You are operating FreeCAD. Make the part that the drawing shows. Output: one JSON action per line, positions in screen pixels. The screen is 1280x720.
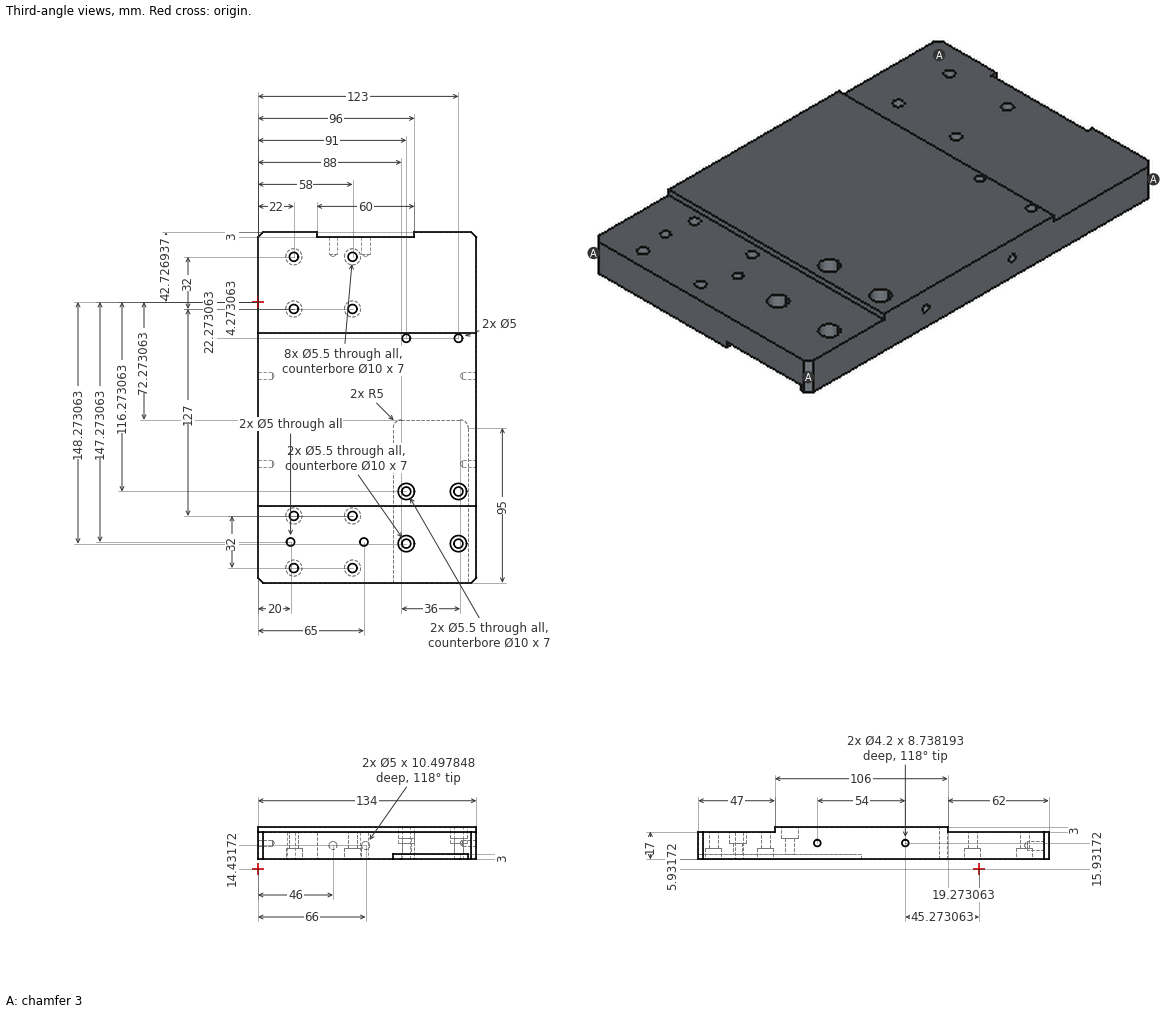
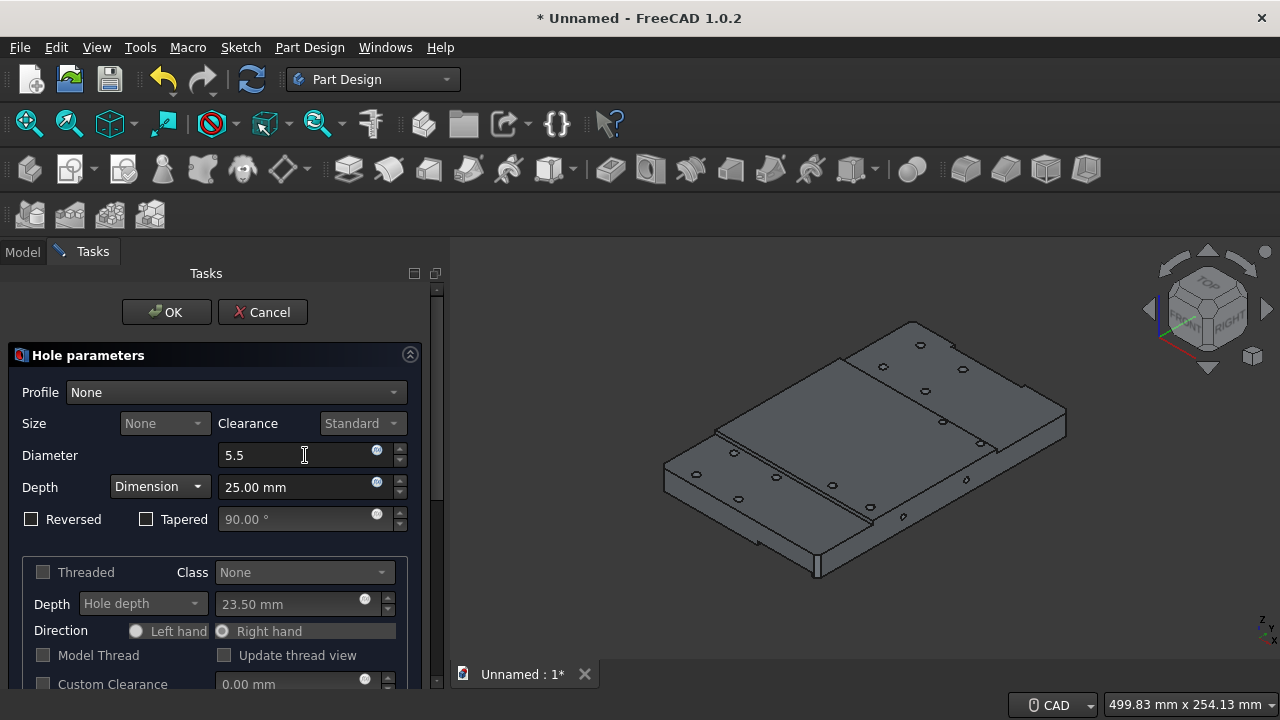
{"action": "left_click", "coordinate": [161, 486]}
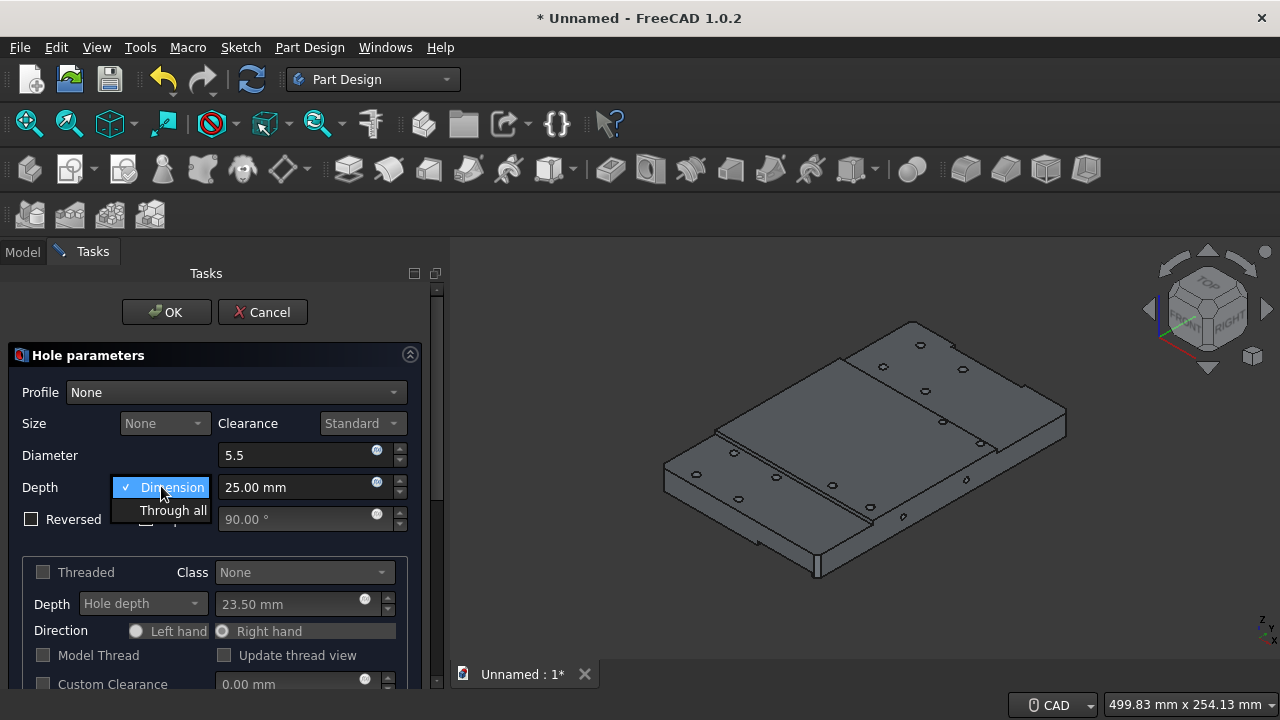
{"action": "left_click", "coordinate": [160, 510]}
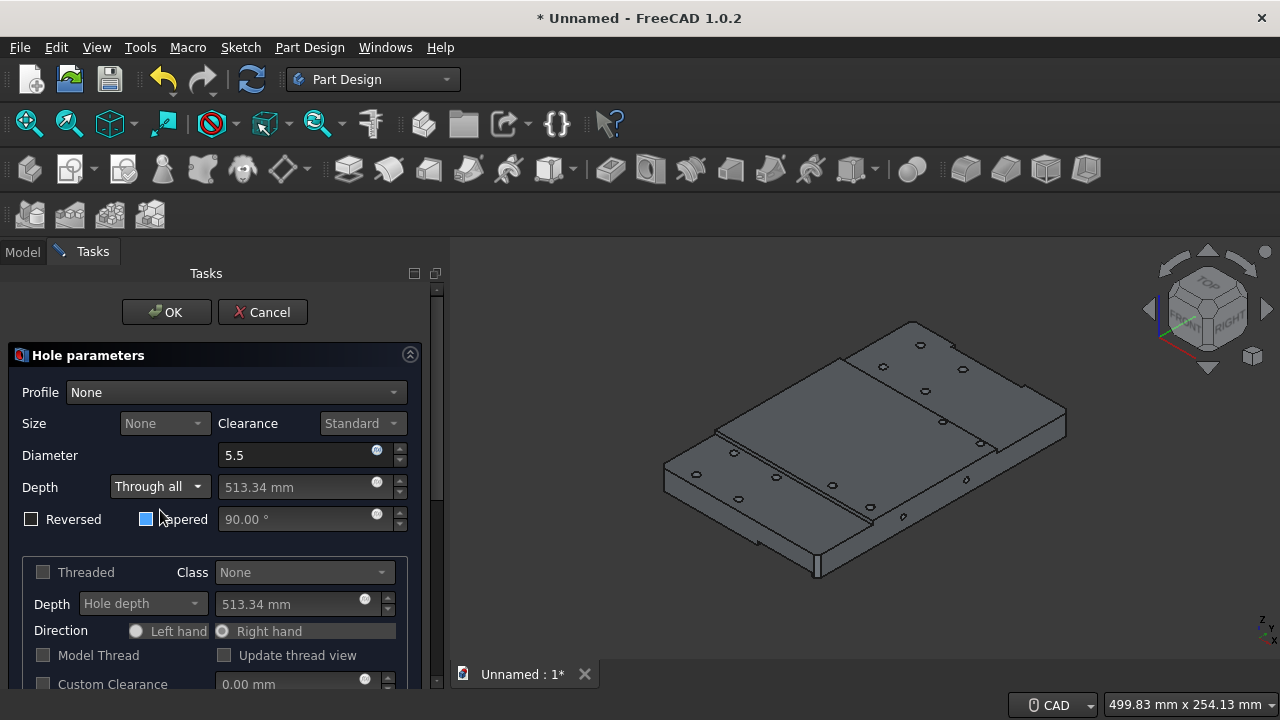
{"action": "scroll", "coordinate": [437, 486], "scroll_direction": "down", "scroll_amount": 3}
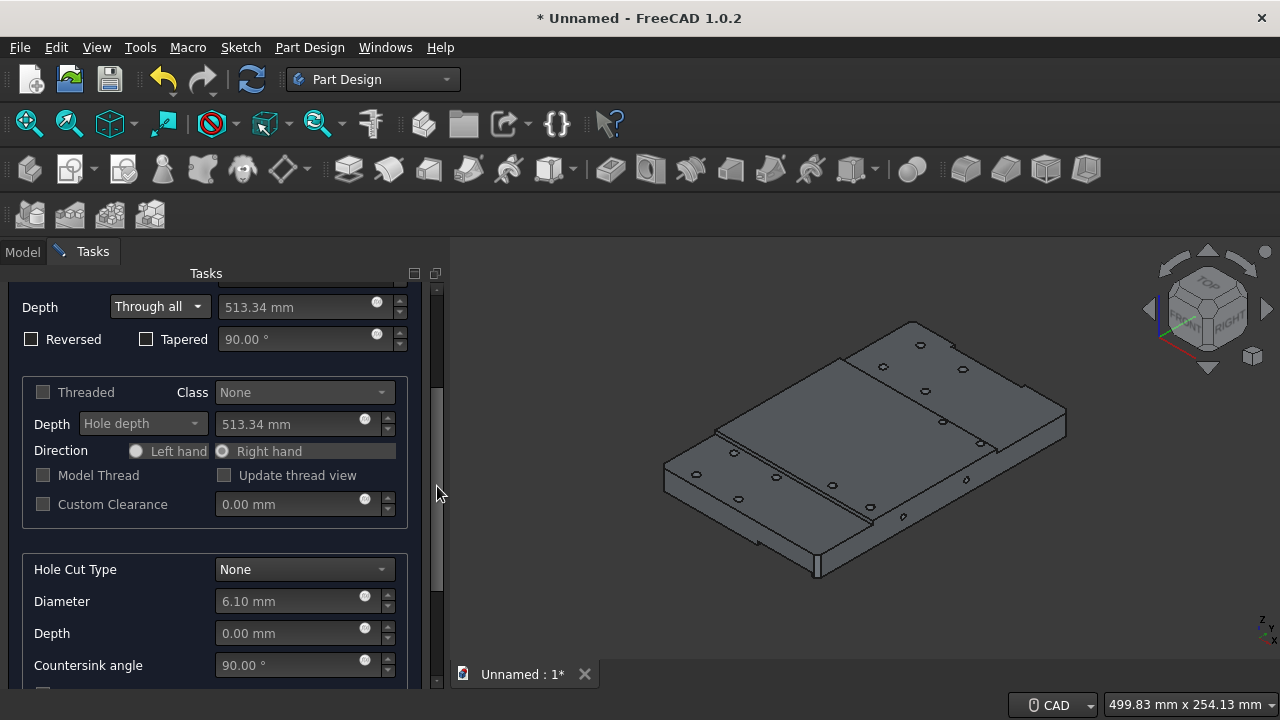
{"action": "left_click", "coordinate": [306, 570]}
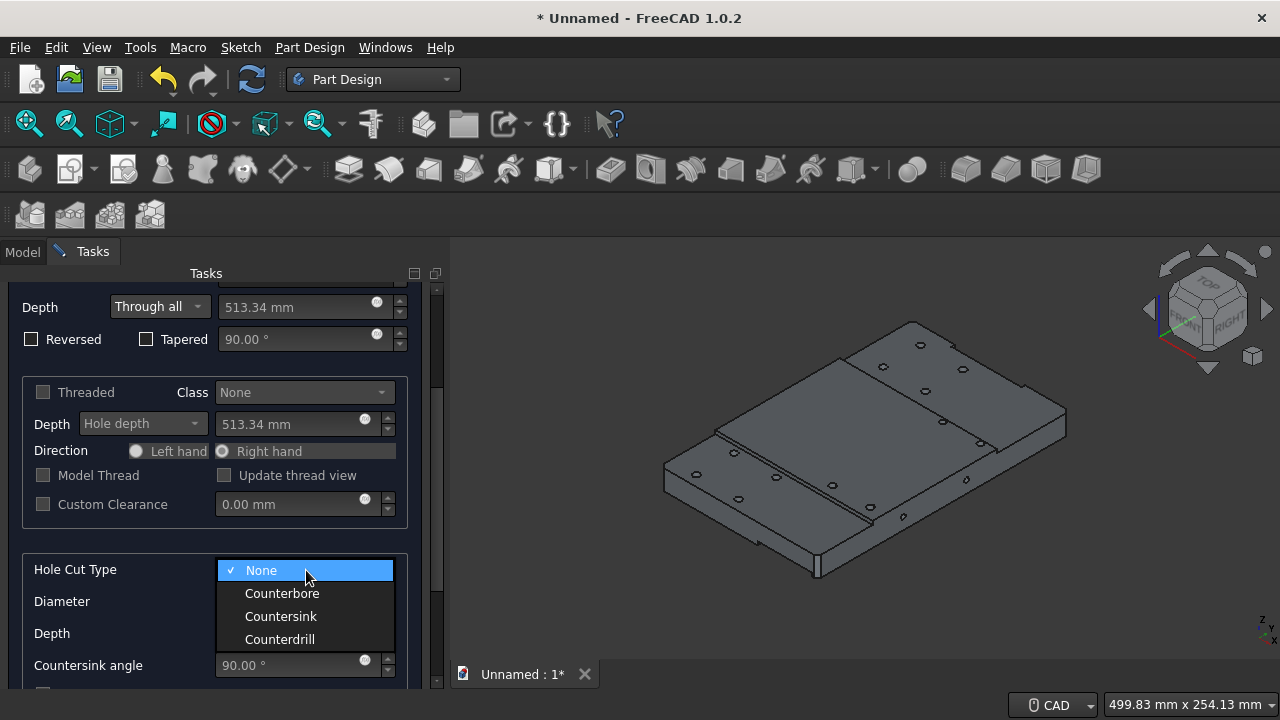
{"action": "left_click", "coordinate": [304, 594]}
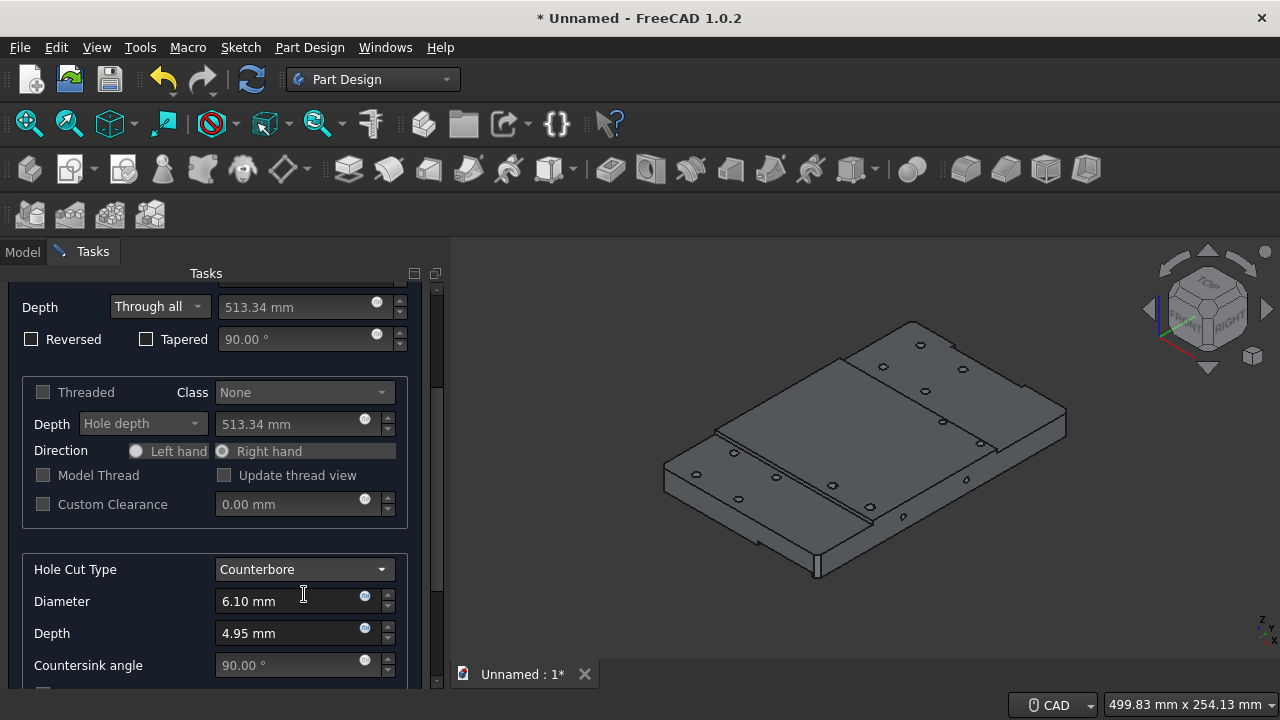
{"action": "triple_click", "coordinate": [298, 601]}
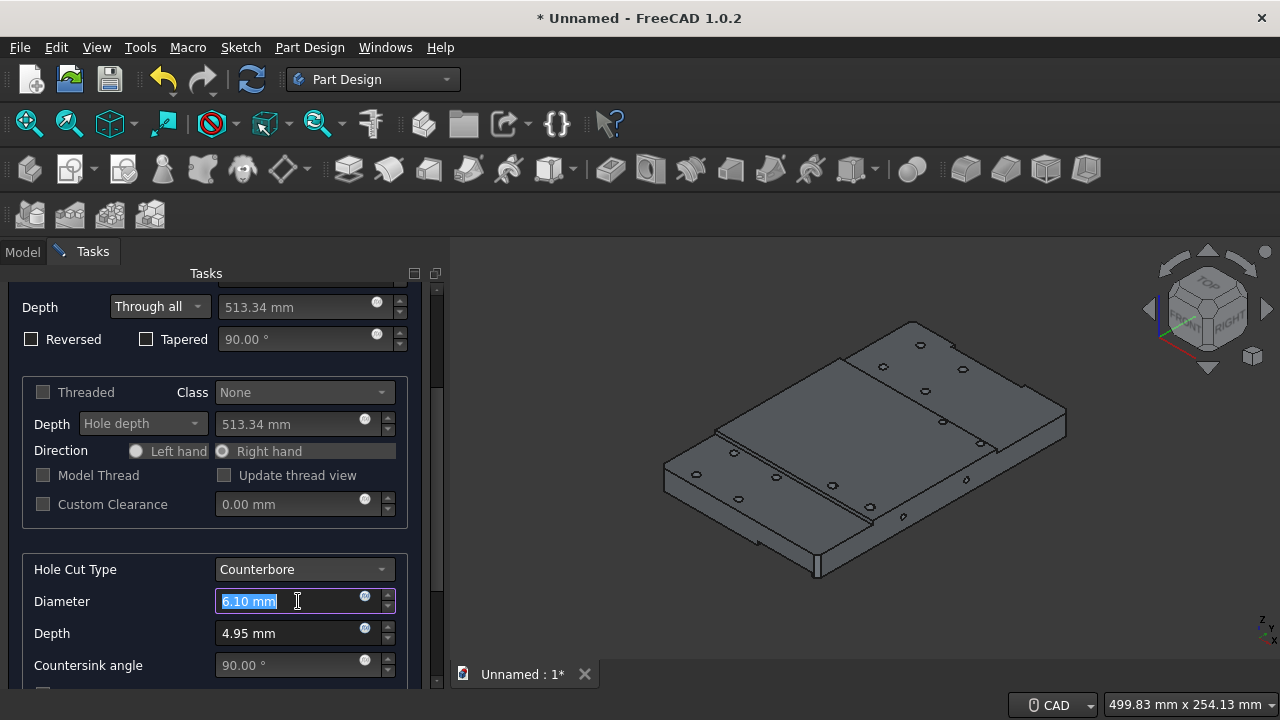
{"action": "type", "text": "10"}
{"action": "key", "text": "Tab"}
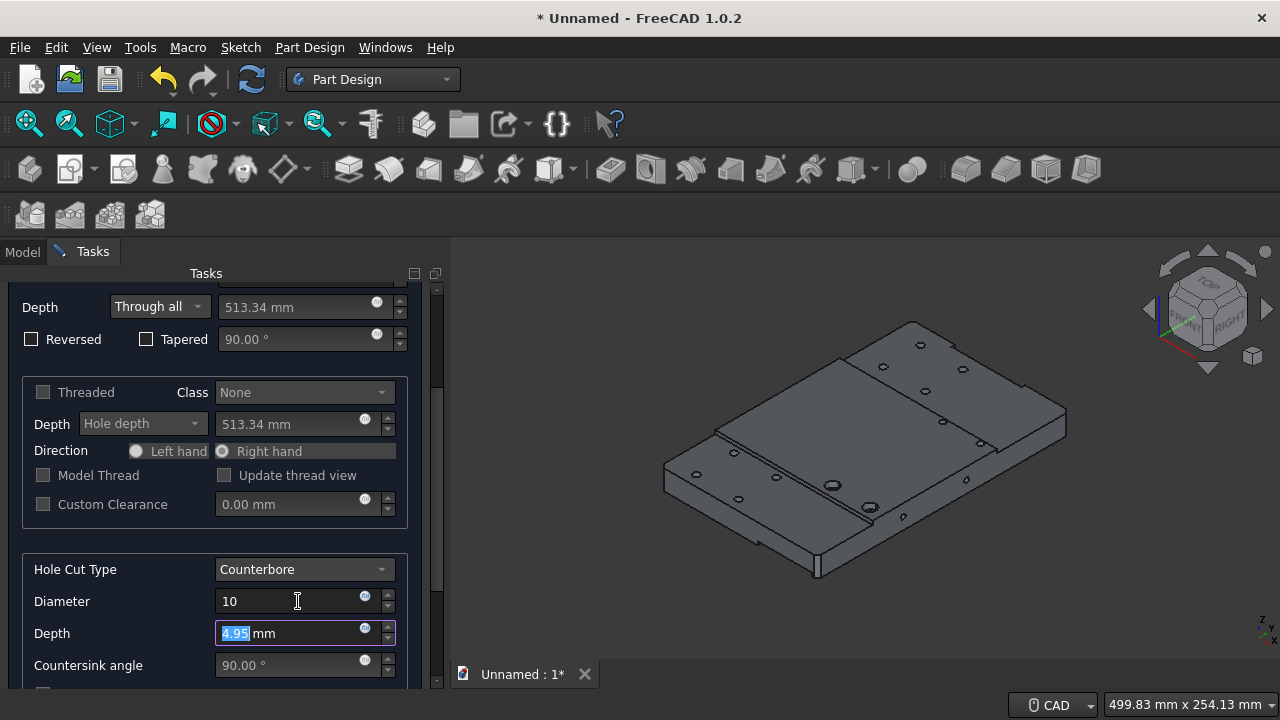
{"action": "type", "text": "7"}
{"action": "key", "text": "Tab"}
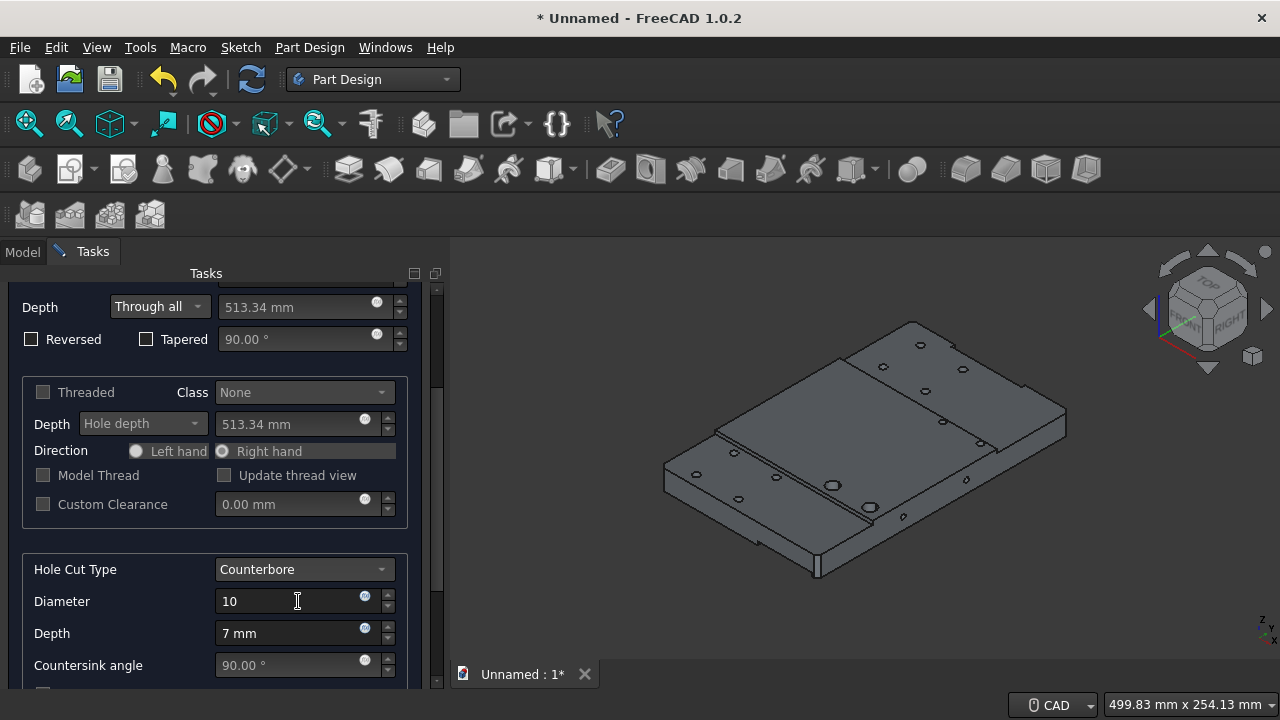
{"action": "scroll", "coordinate": [437, 486], "scroll_direction": "up", "scroll_amount": 4}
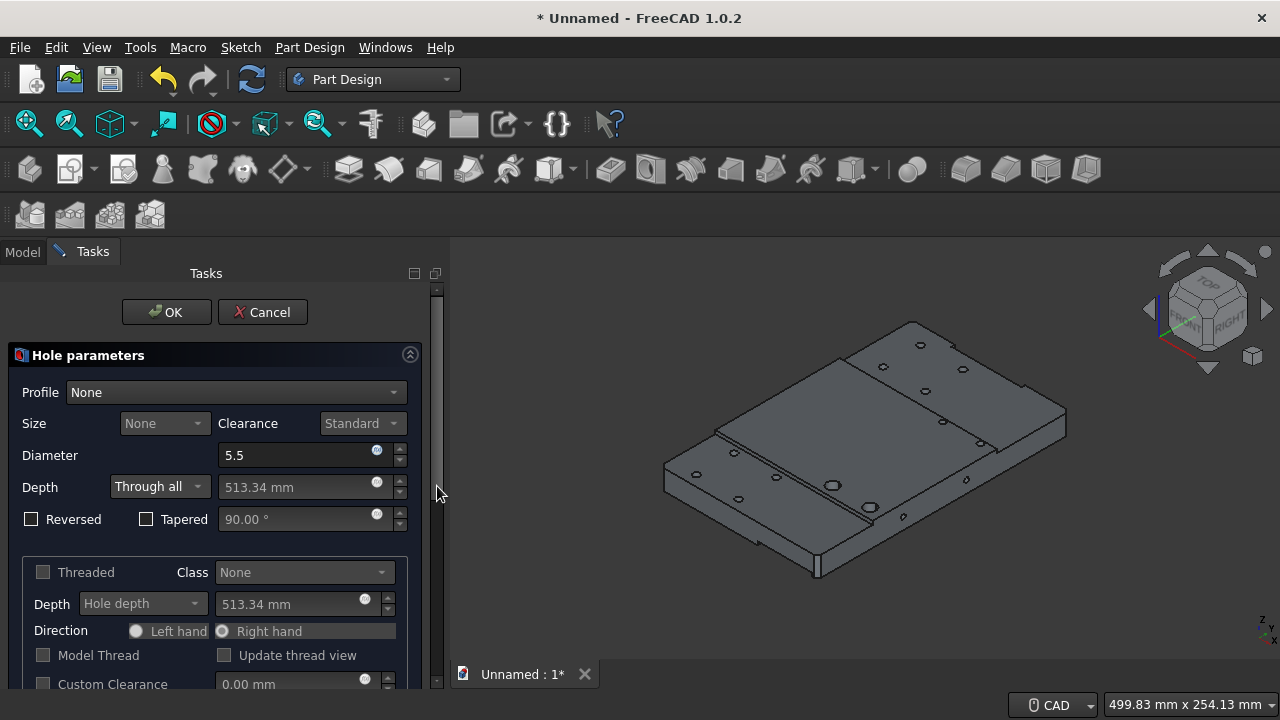
{"action": "left_click", "coordinate": [167, 312]}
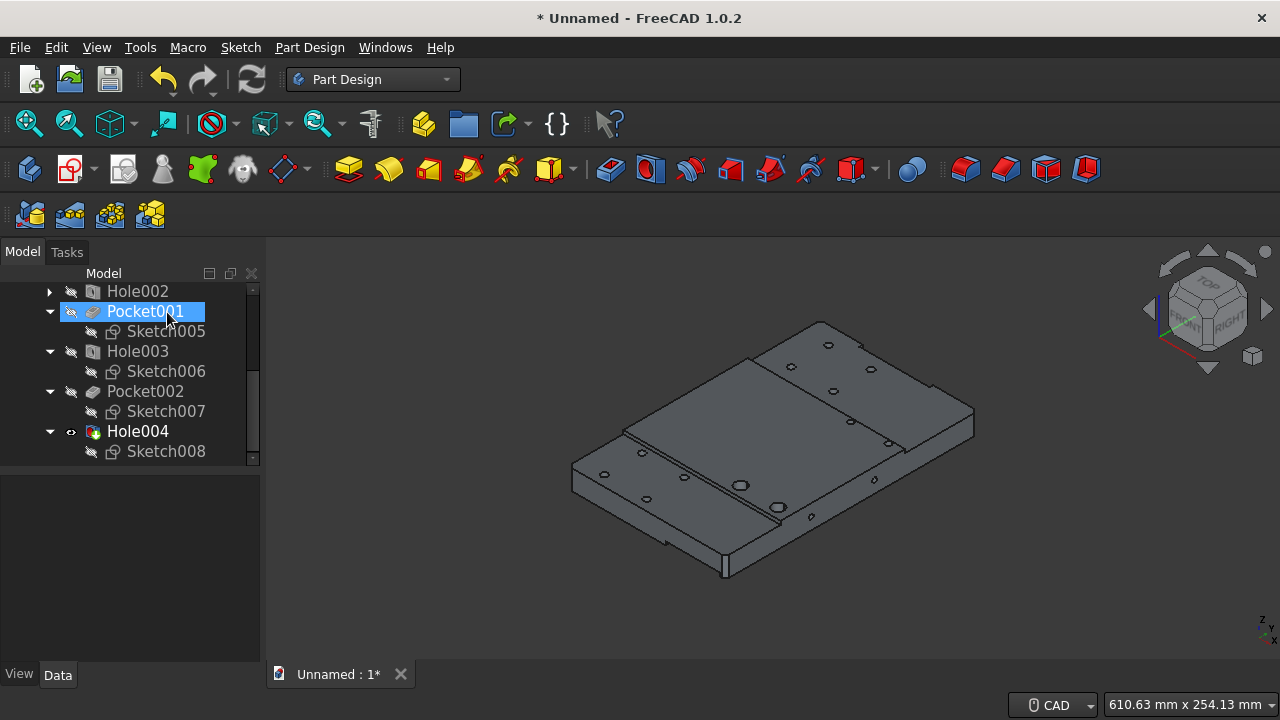
{"action": "left_click", "coordinate": [908, 412]}